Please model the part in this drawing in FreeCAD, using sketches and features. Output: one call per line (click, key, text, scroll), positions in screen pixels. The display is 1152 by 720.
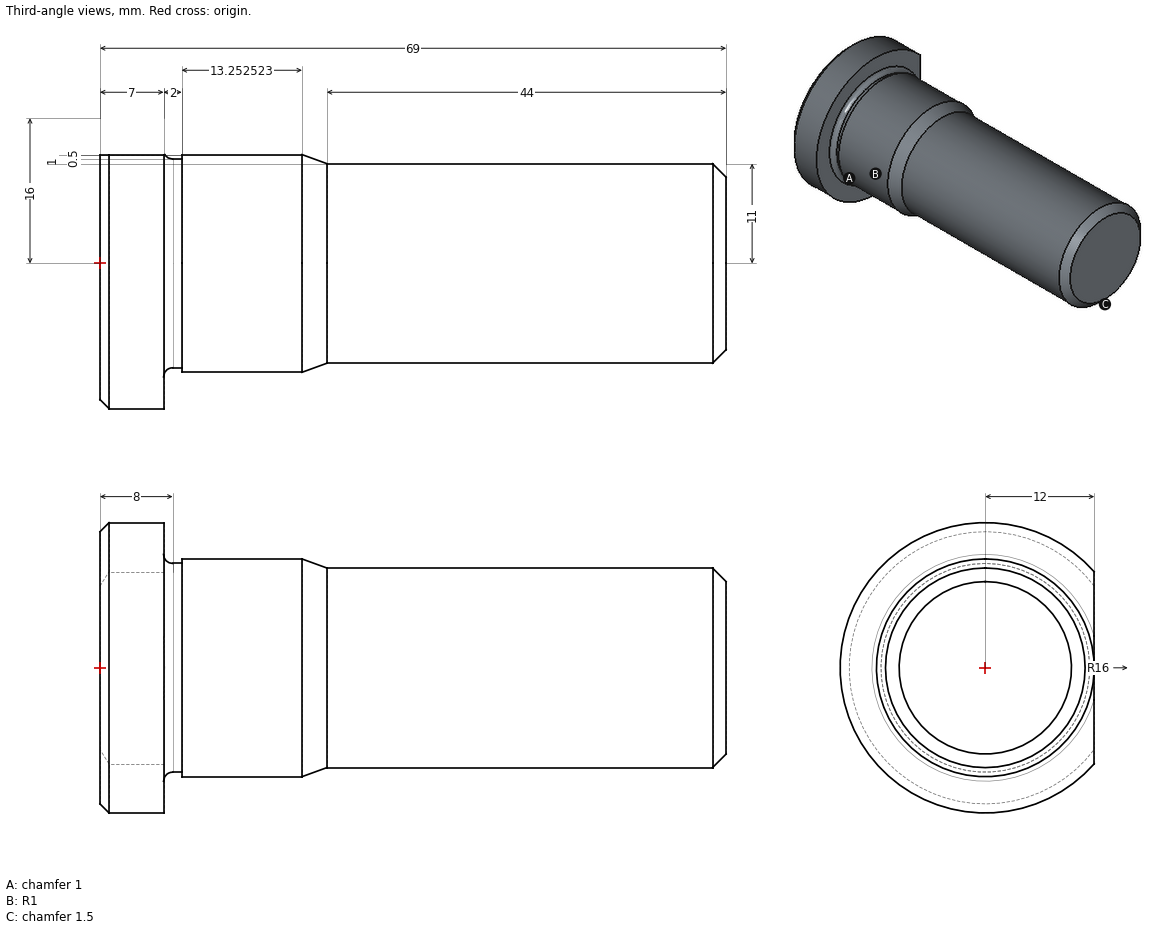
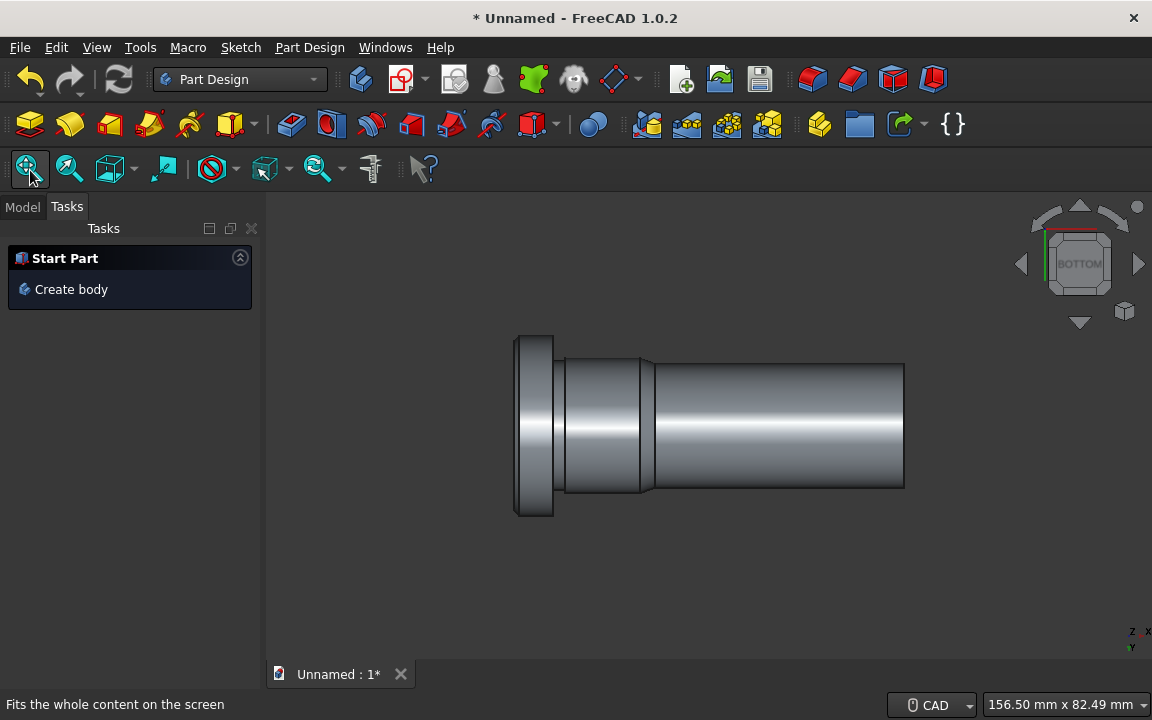
click(30, 170)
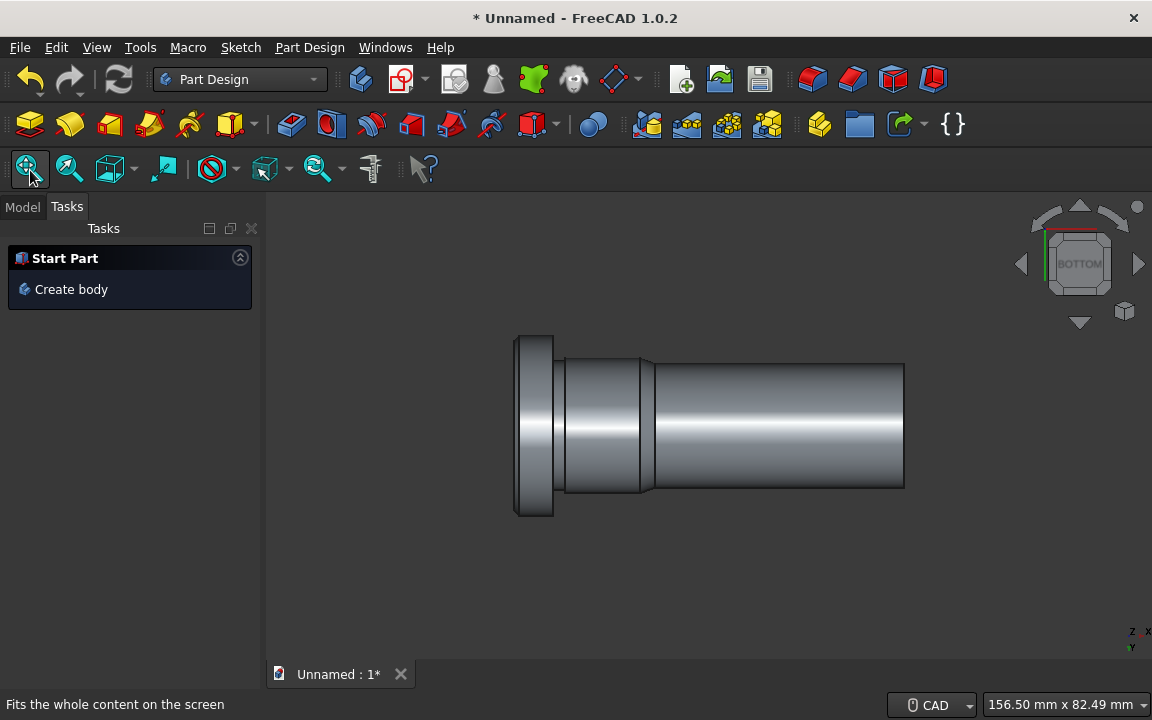
key(4)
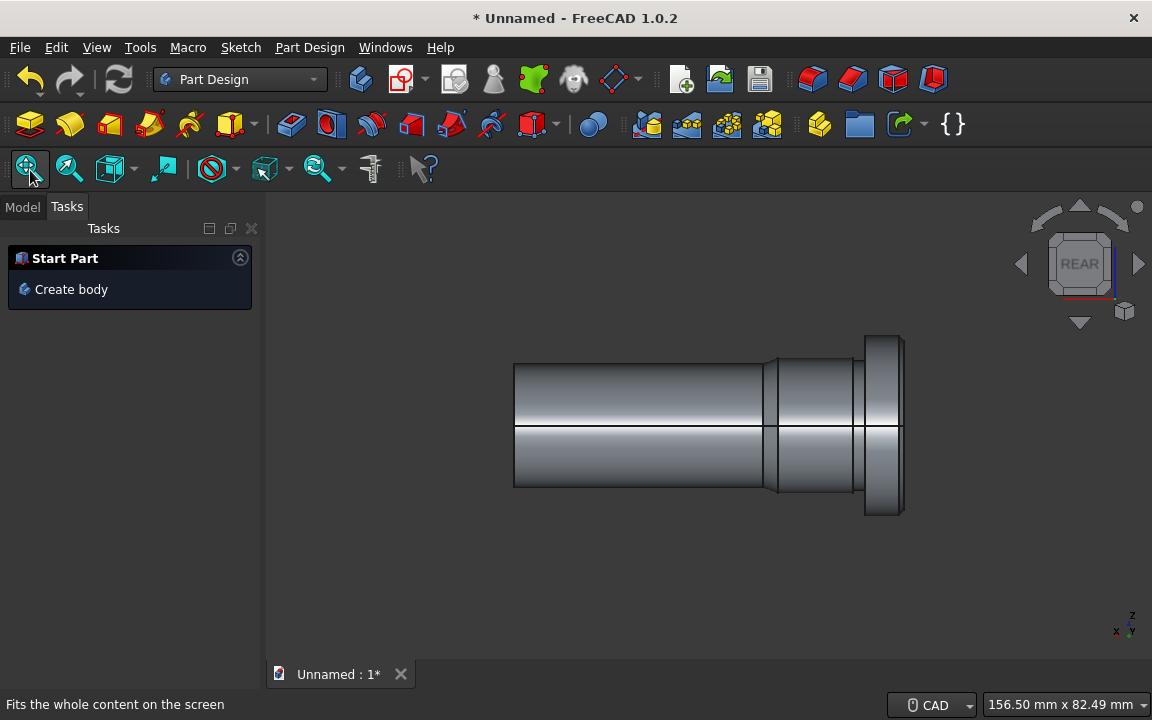
click(30, 170)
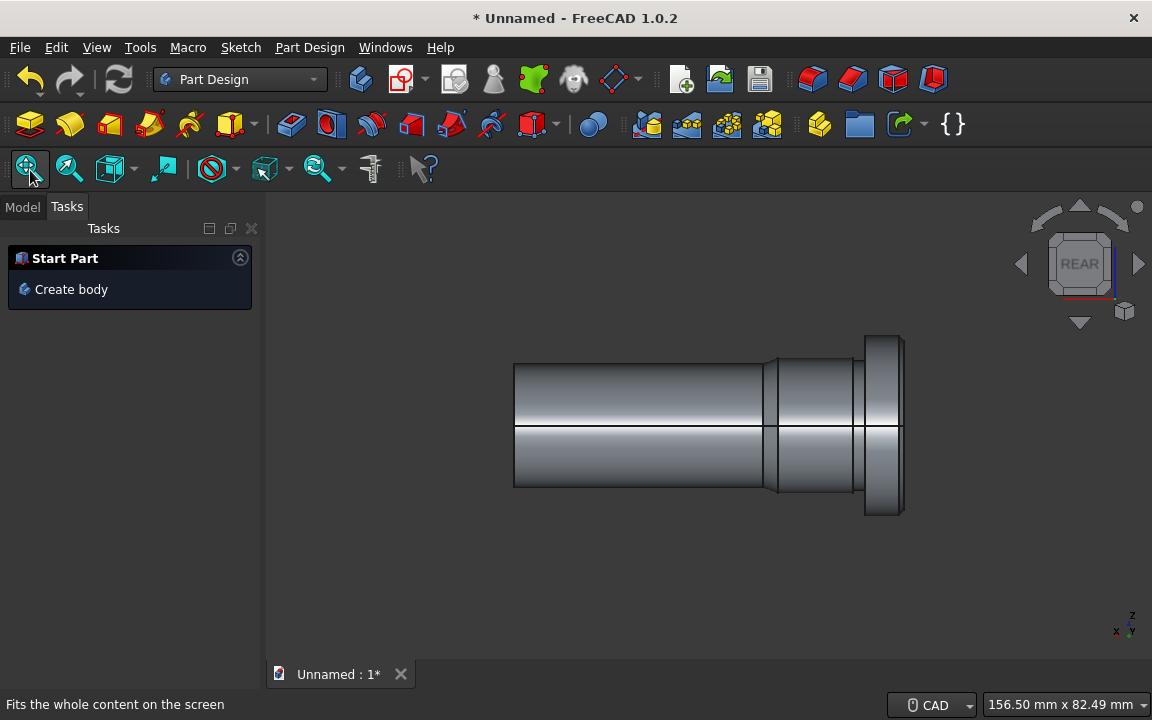
key(6)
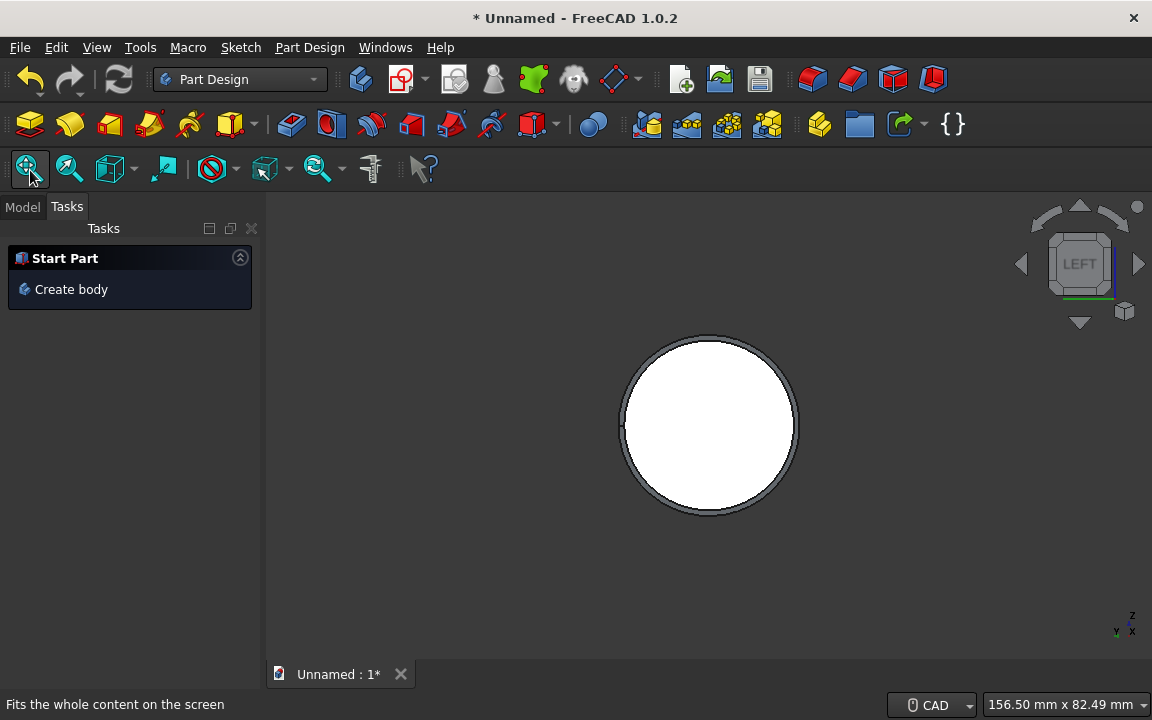
click(30, 170)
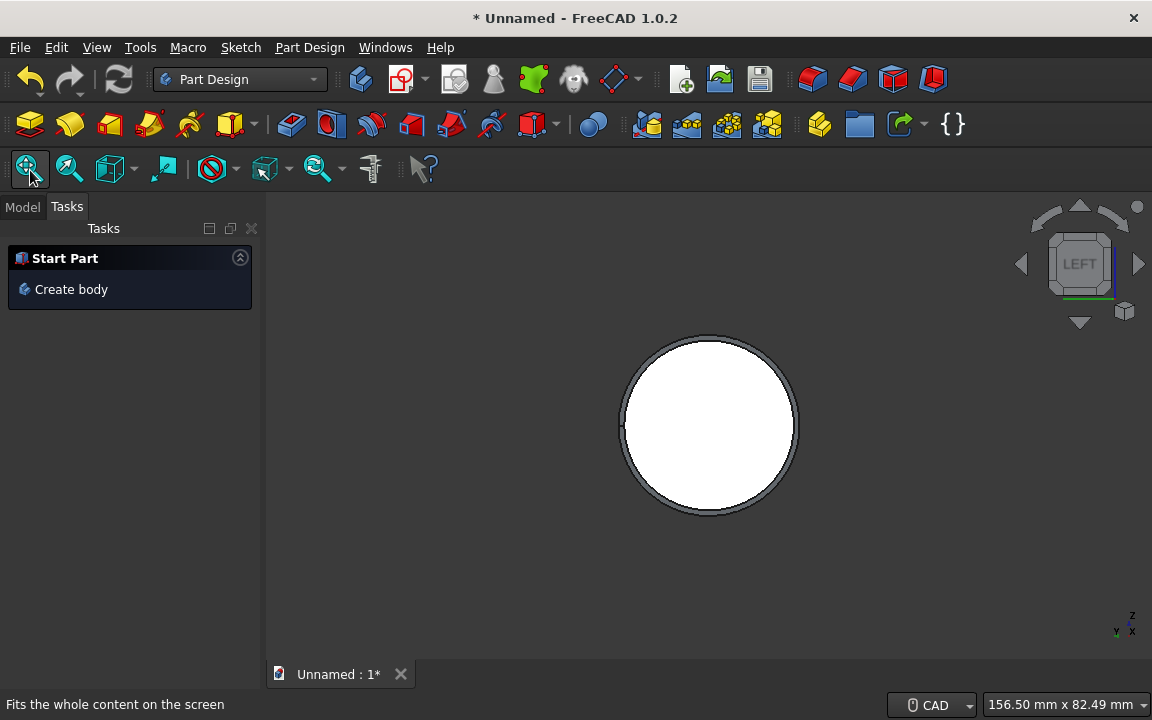
key(v)
key(3)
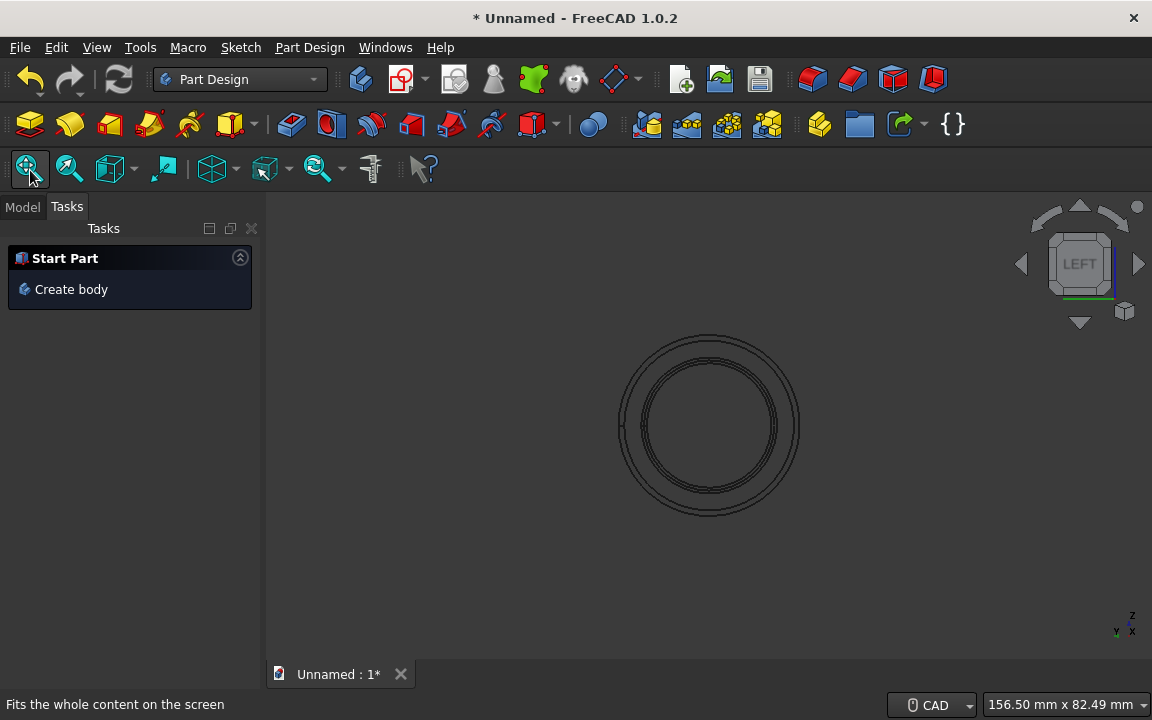
key(0)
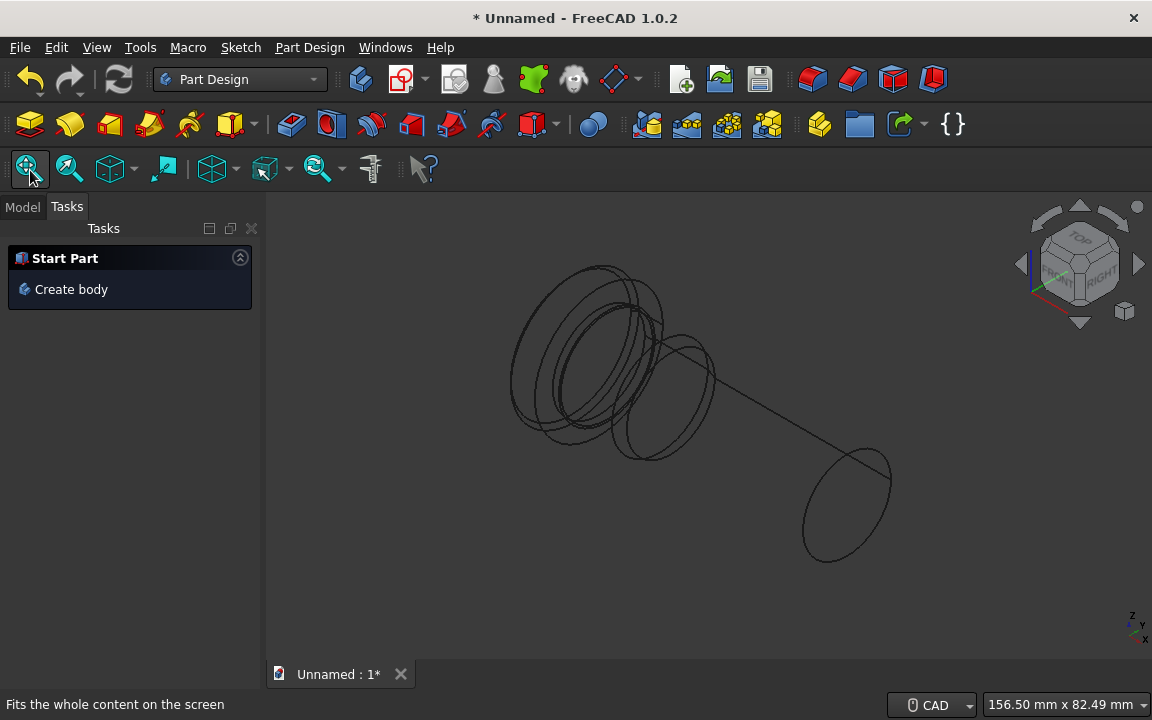
click(562, 351)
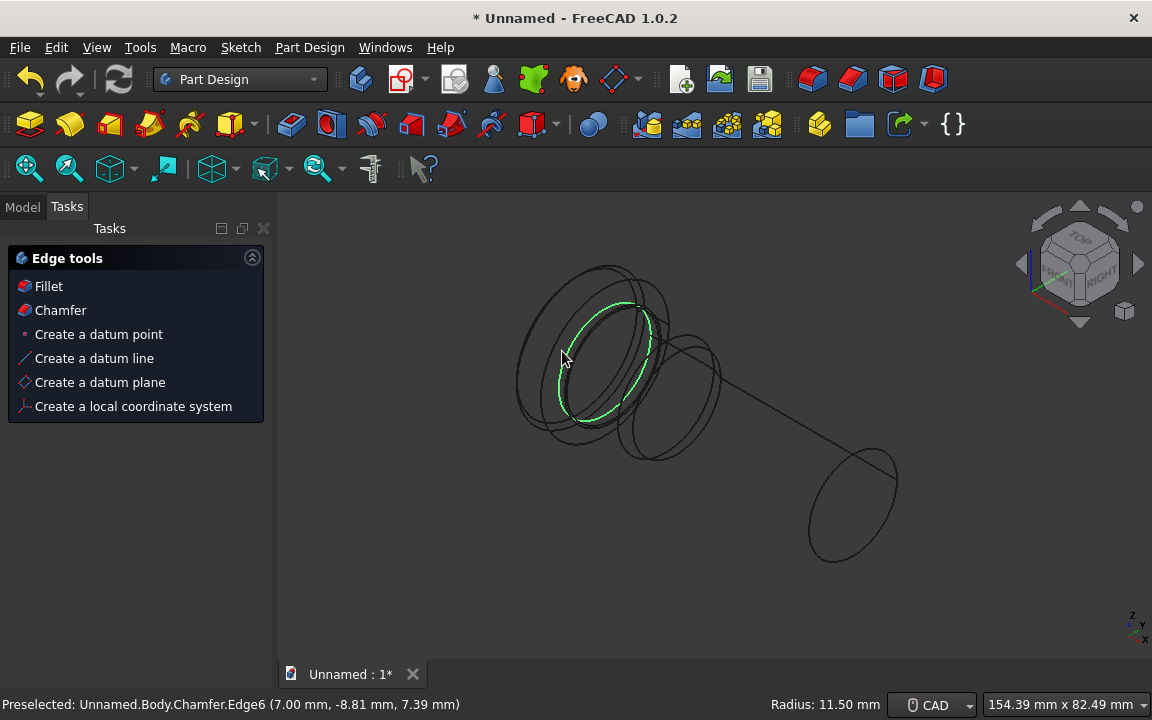
key(v)
key(1)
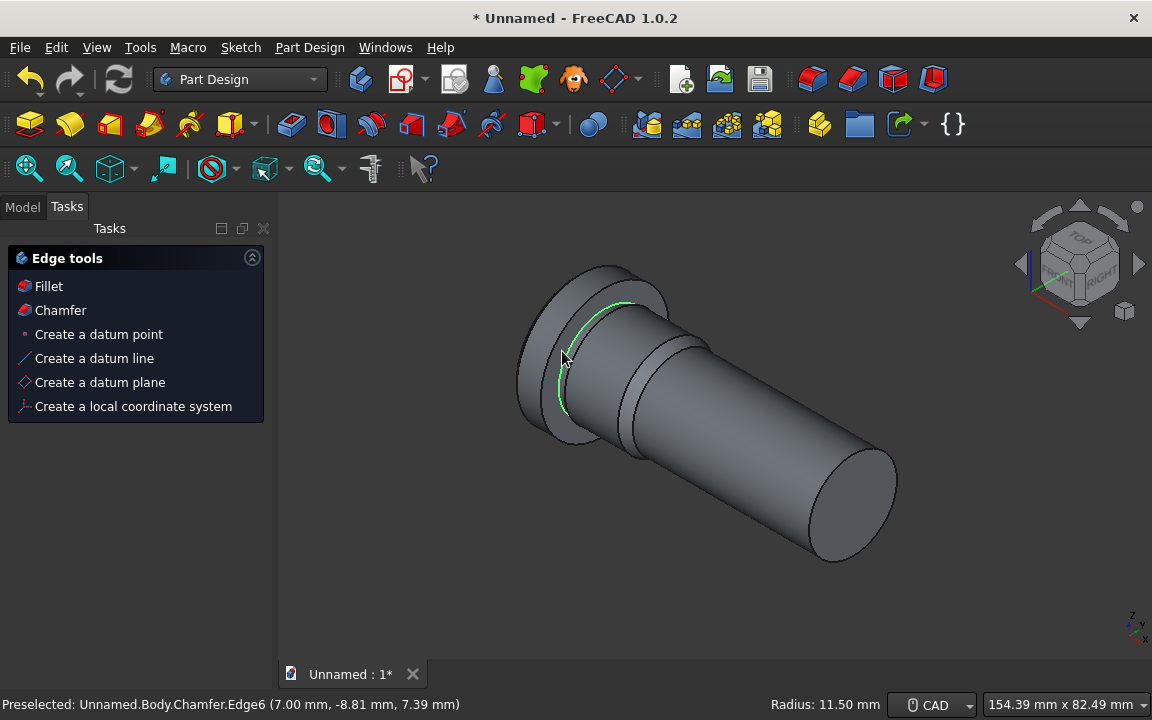
click(814, 80)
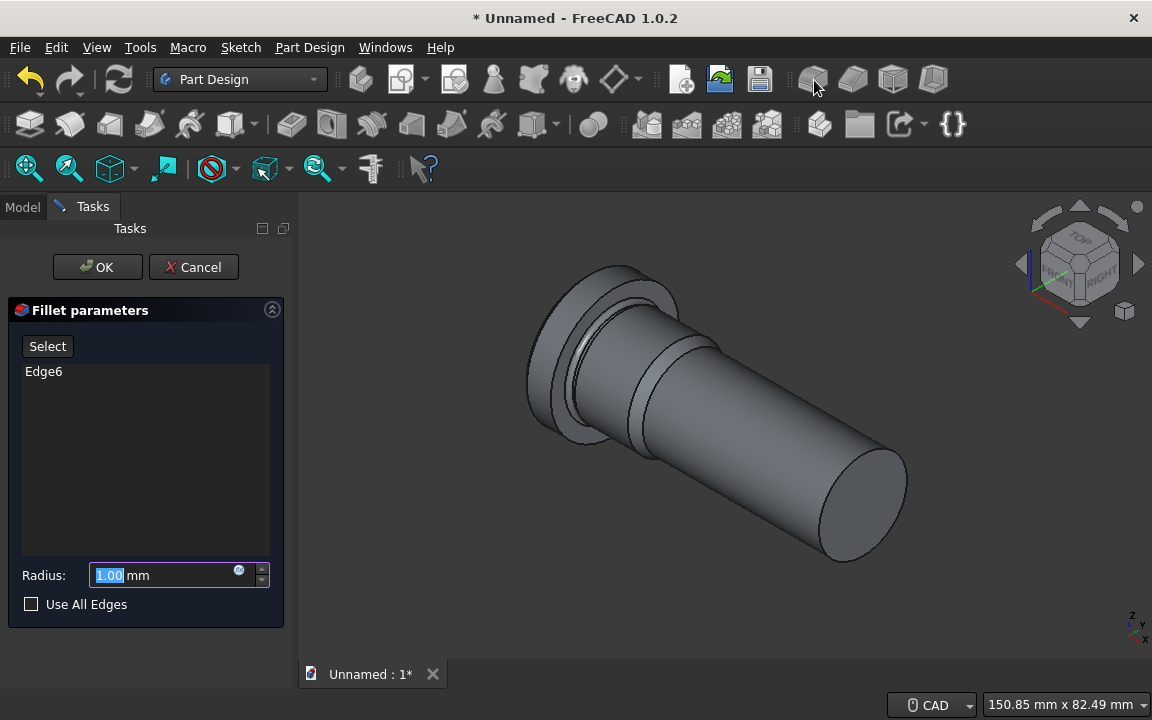
text(1)
key(Tab)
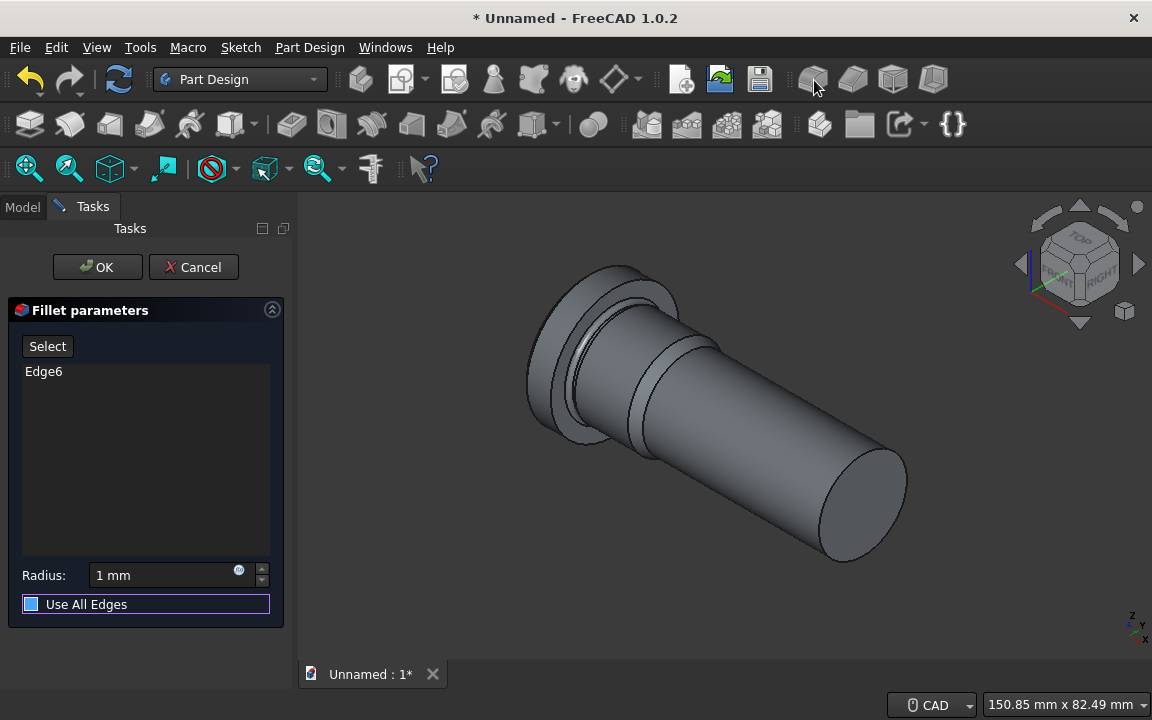
click(98, 267)